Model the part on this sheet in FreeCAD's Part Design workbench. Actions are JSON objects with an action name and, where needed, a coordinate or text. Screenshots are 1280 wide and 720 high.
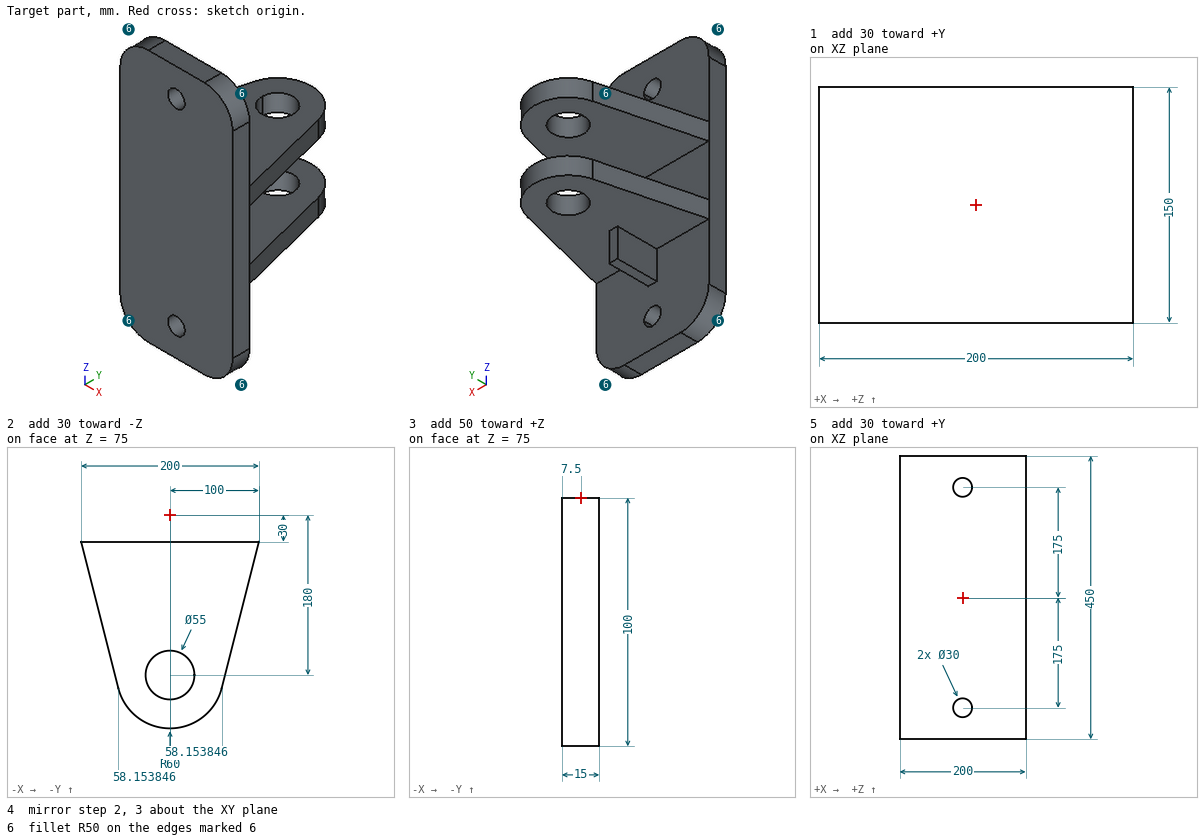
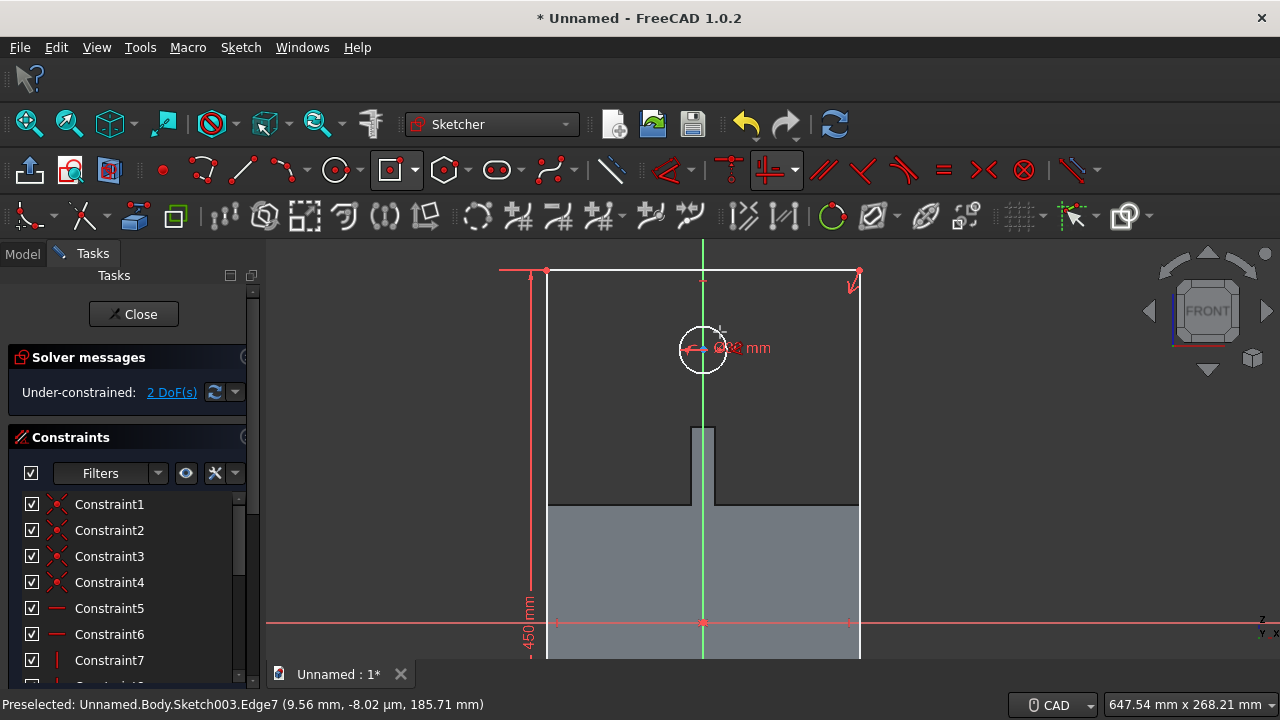
{"action": "scroll", "coordinate": [705, 348], "scroll_direction": "down", "scroll_amount": 5}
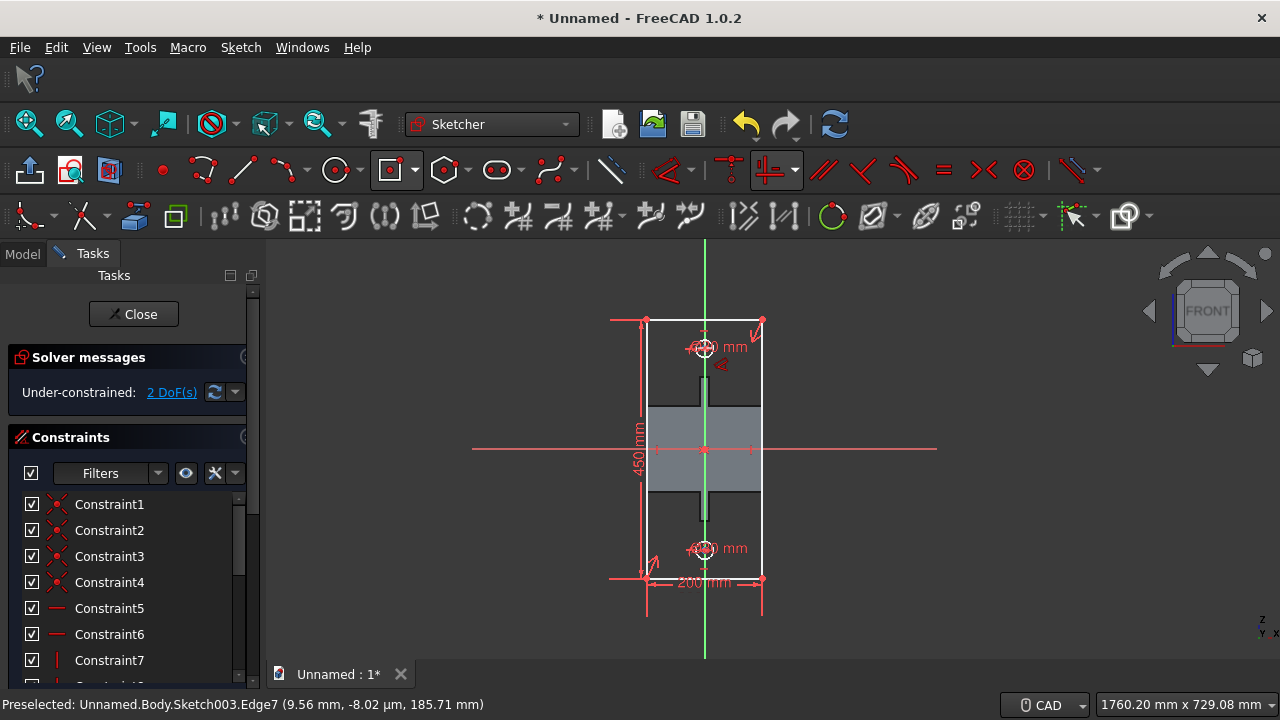
{"action": "left_click", "coordinate": [705, 550]}
{"action": "left_click", "coordinate": [739, 500]}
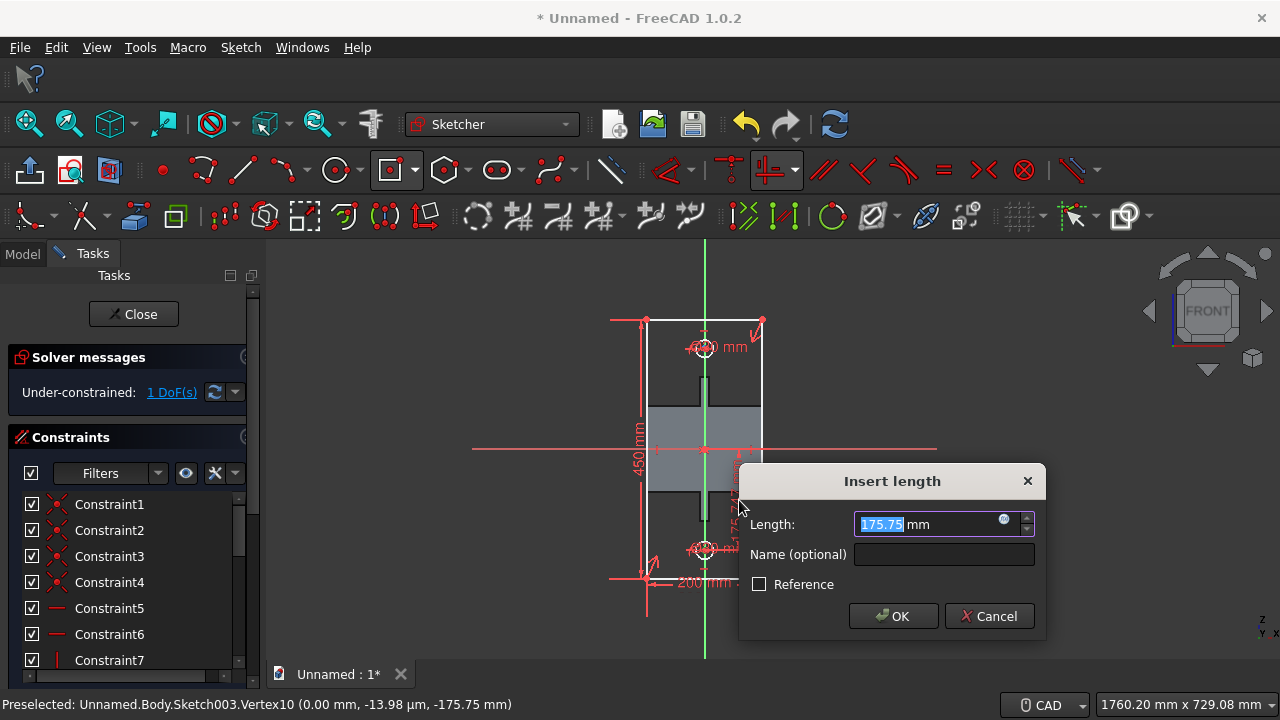
{"action": "type", "text": "175"}
{"action": "key", "text": "Return"}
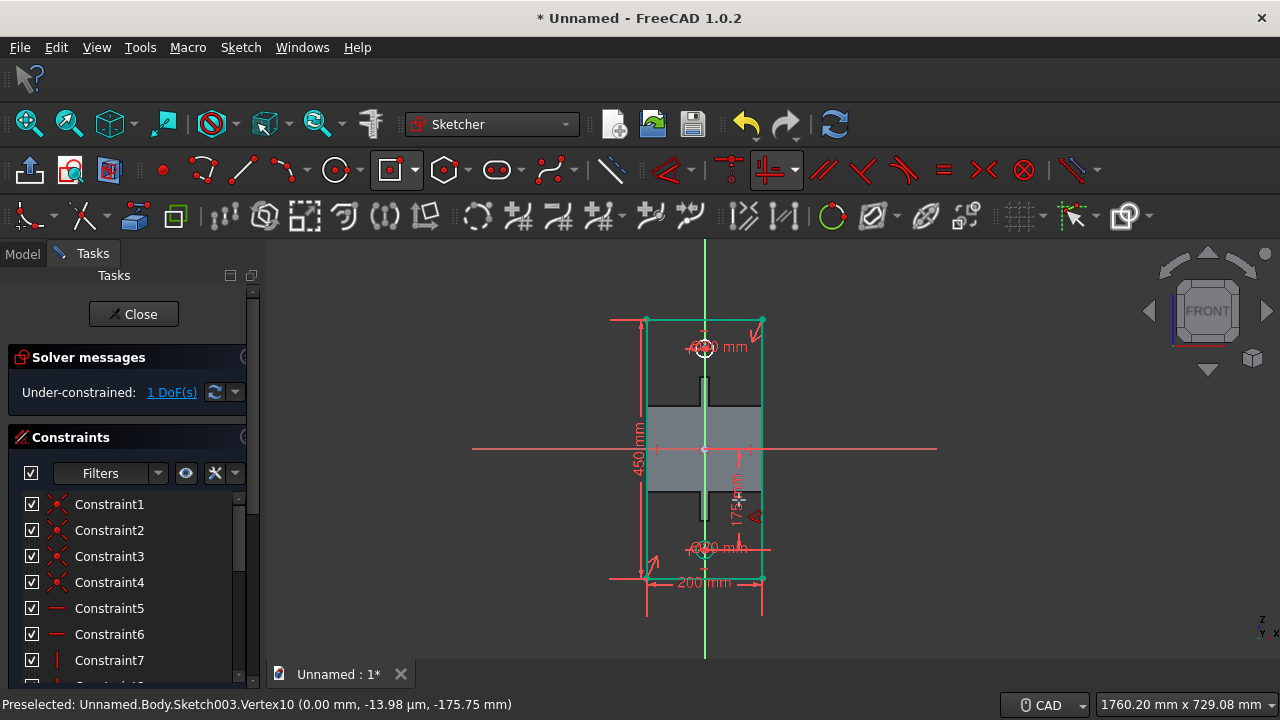
{"action": "left_click", "coordinate": [705, 349]}
{"action": "left_click", "coordinate": [739, 399]}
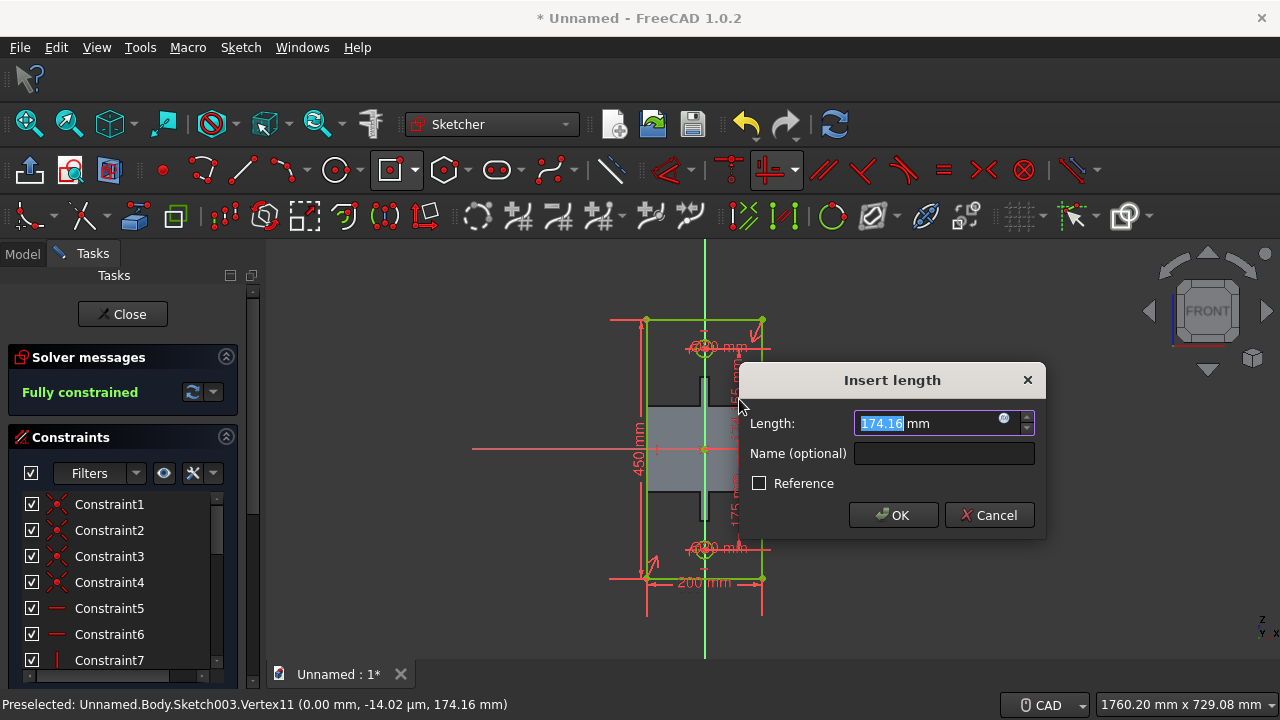
{"action": "type", "text": "175"}
{"action": "key", "text": "Return"}
{"action": "key", "text": "Escape"}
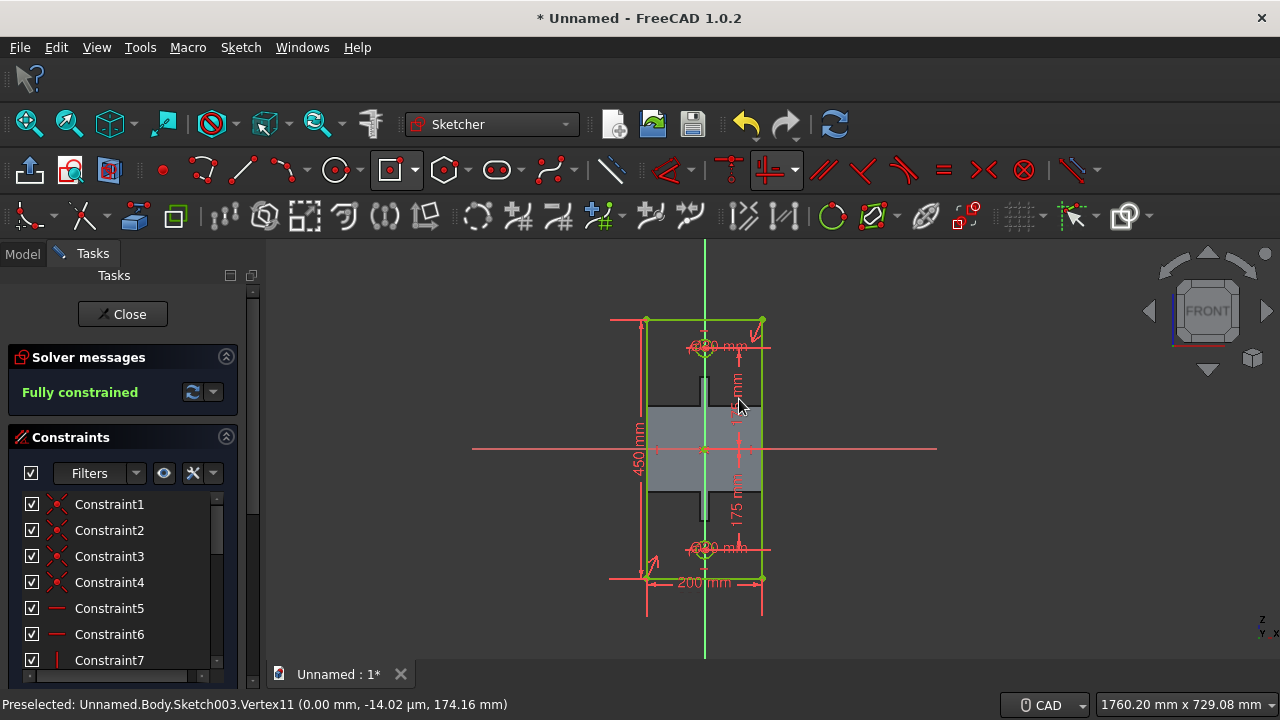
{"action": "left_click", "coordinate": [123, 314]}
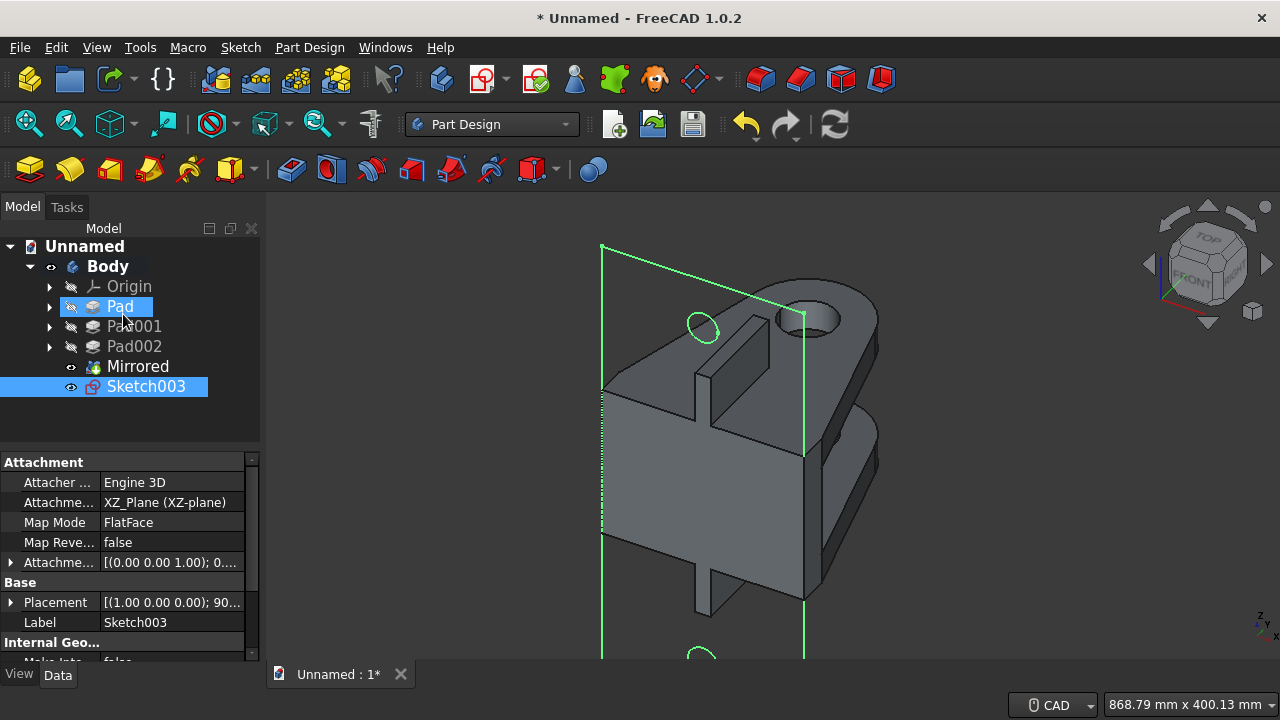
{"action": "left_click", "coordinate": [30, 170]}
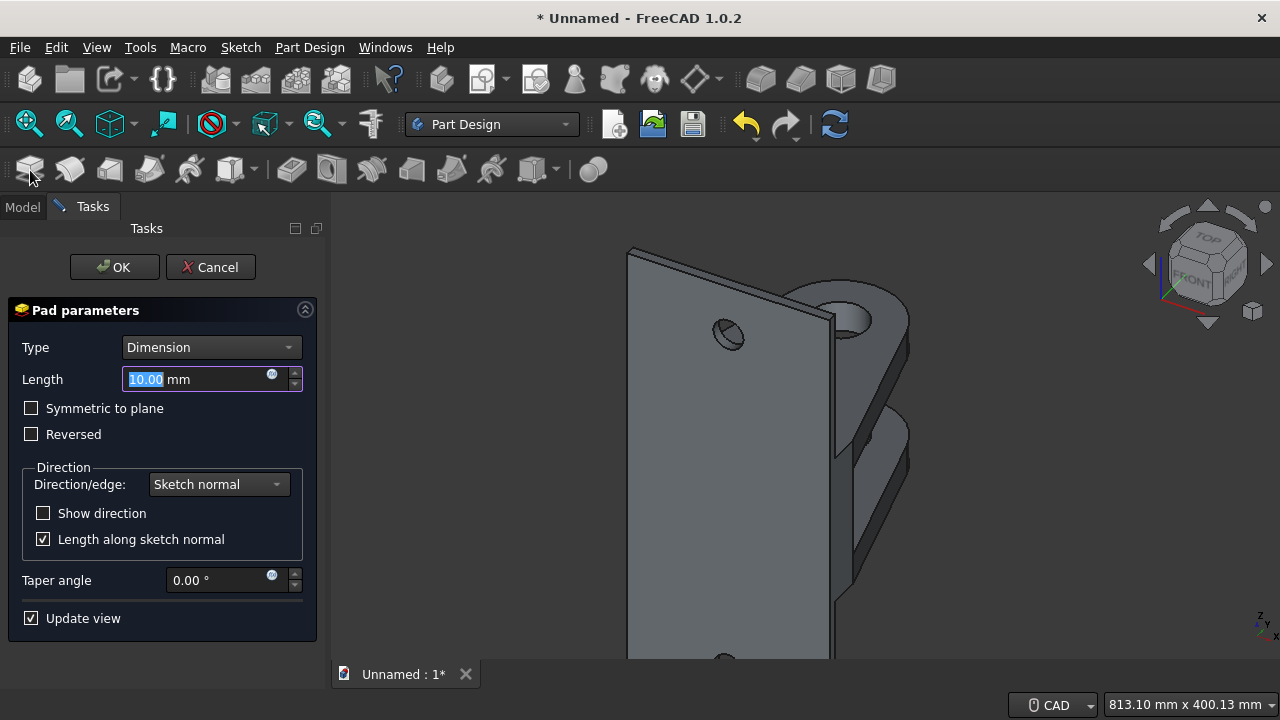
{"action": "type", "text": "30"}
{"action": "key", "text": "Tab"}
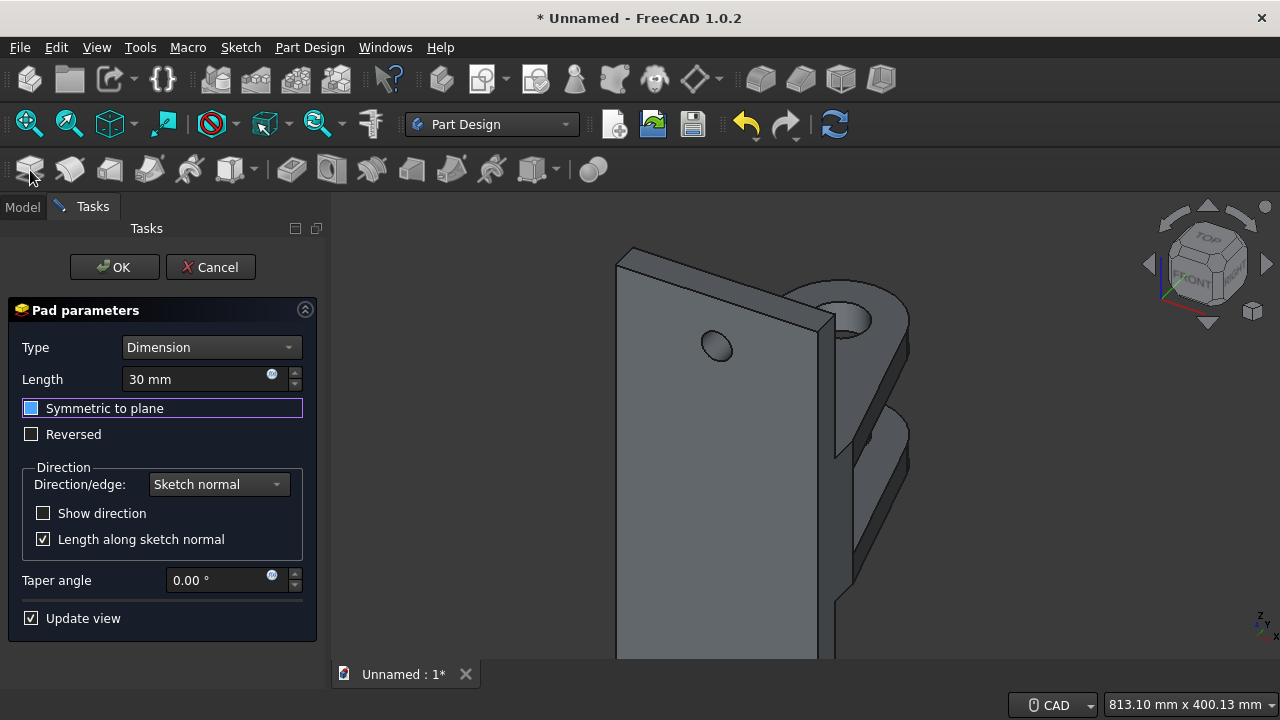
{"action": "left_click", "coordinate": [30, 434]}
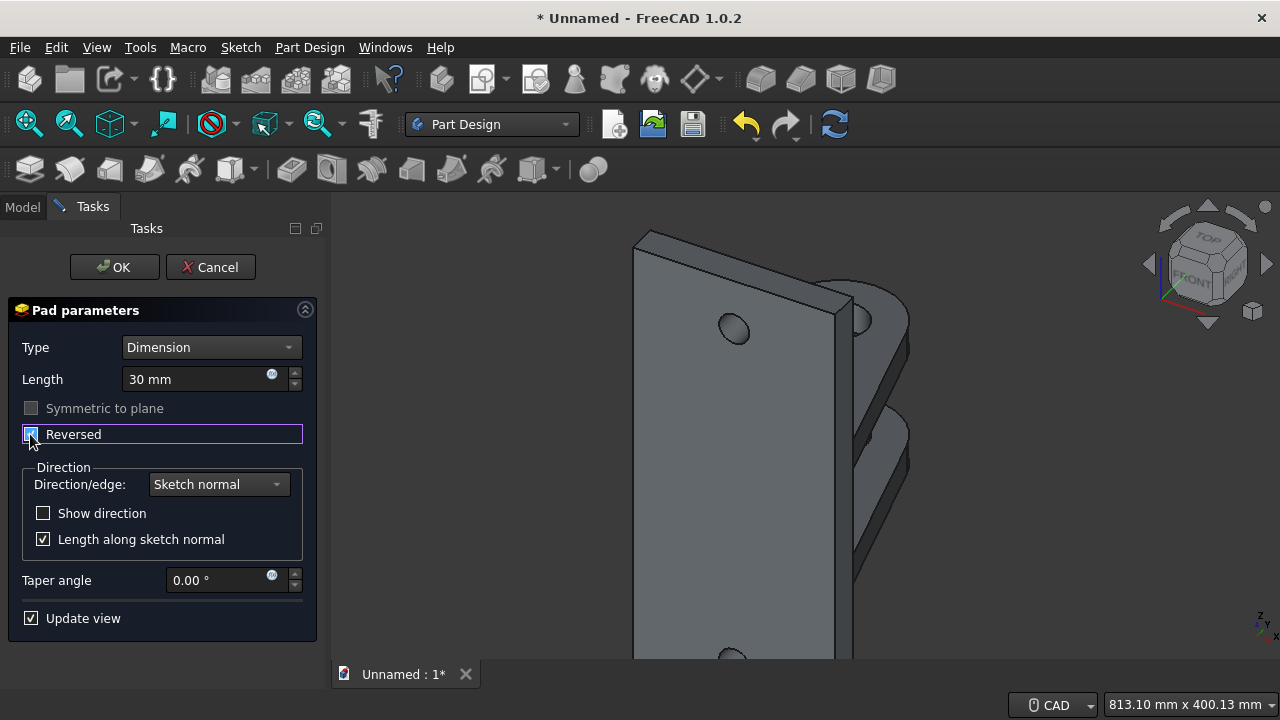
{"action": "left_click", "coordinate": [115, 267]}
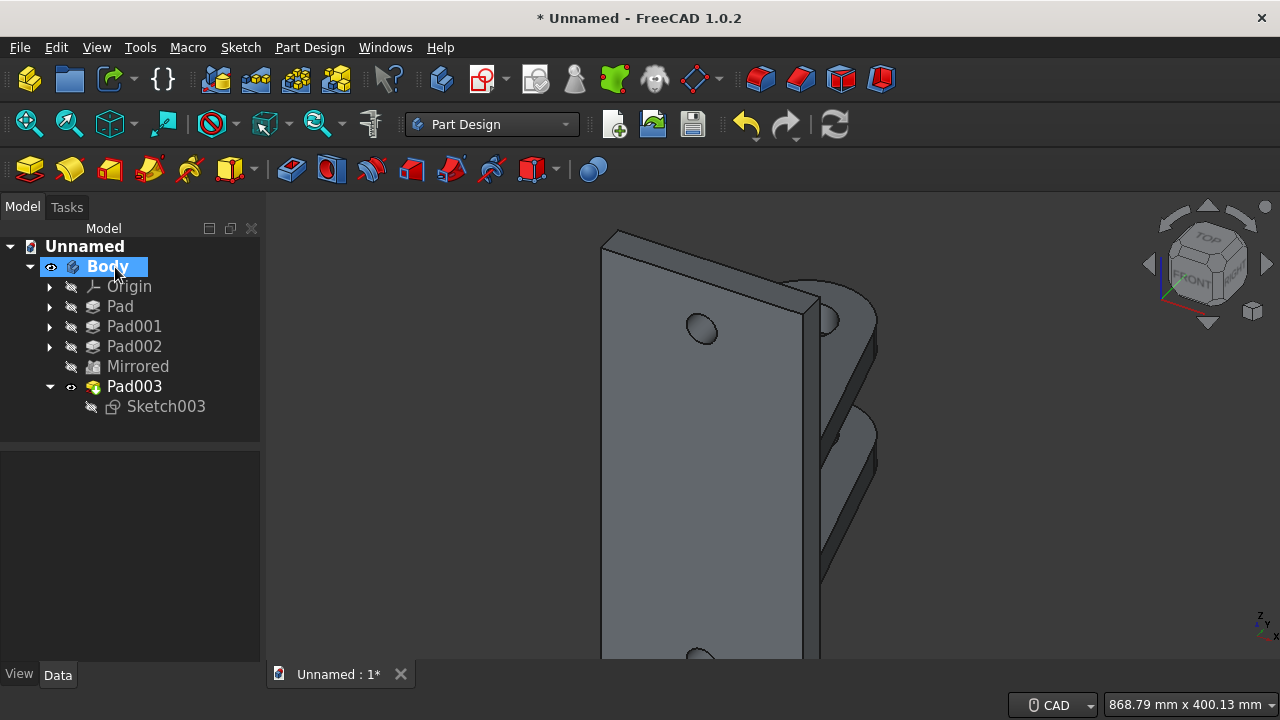
{"action": "left_click", "coordinate": [30, 124]}